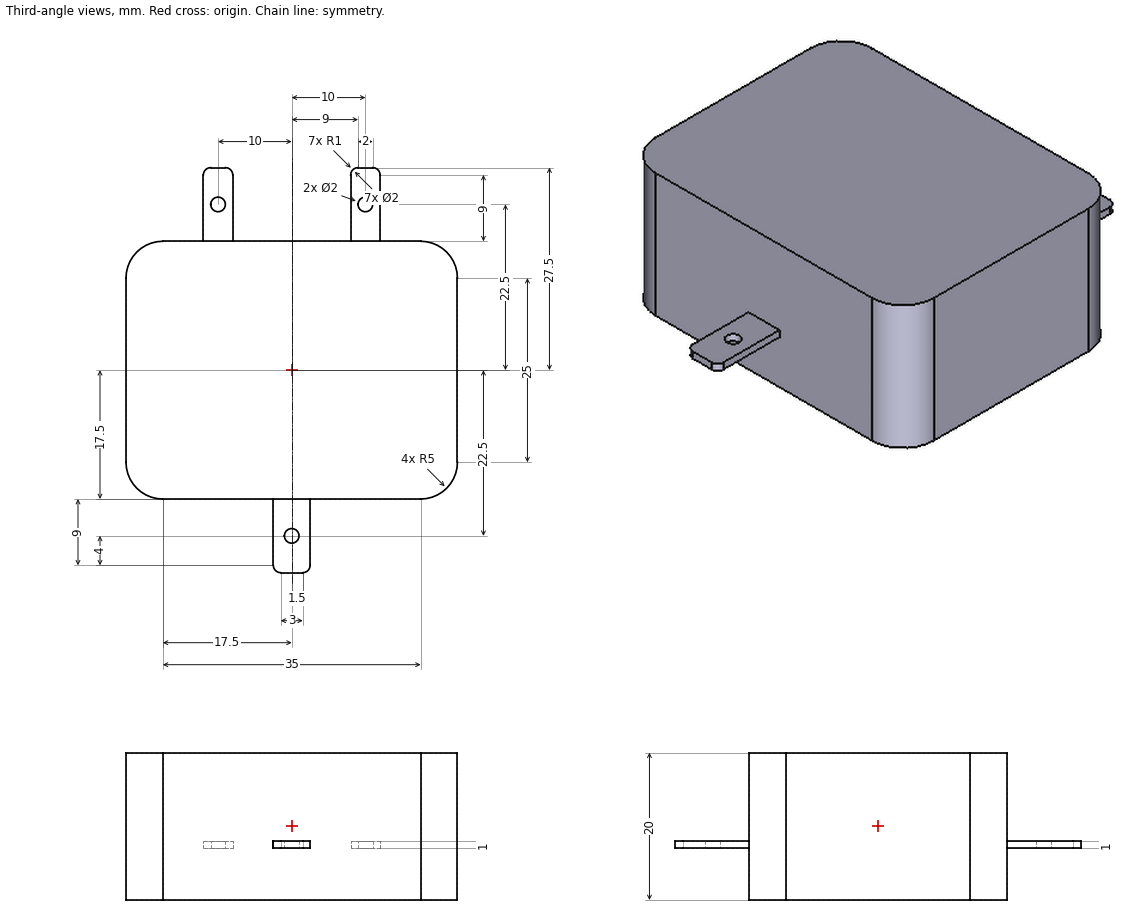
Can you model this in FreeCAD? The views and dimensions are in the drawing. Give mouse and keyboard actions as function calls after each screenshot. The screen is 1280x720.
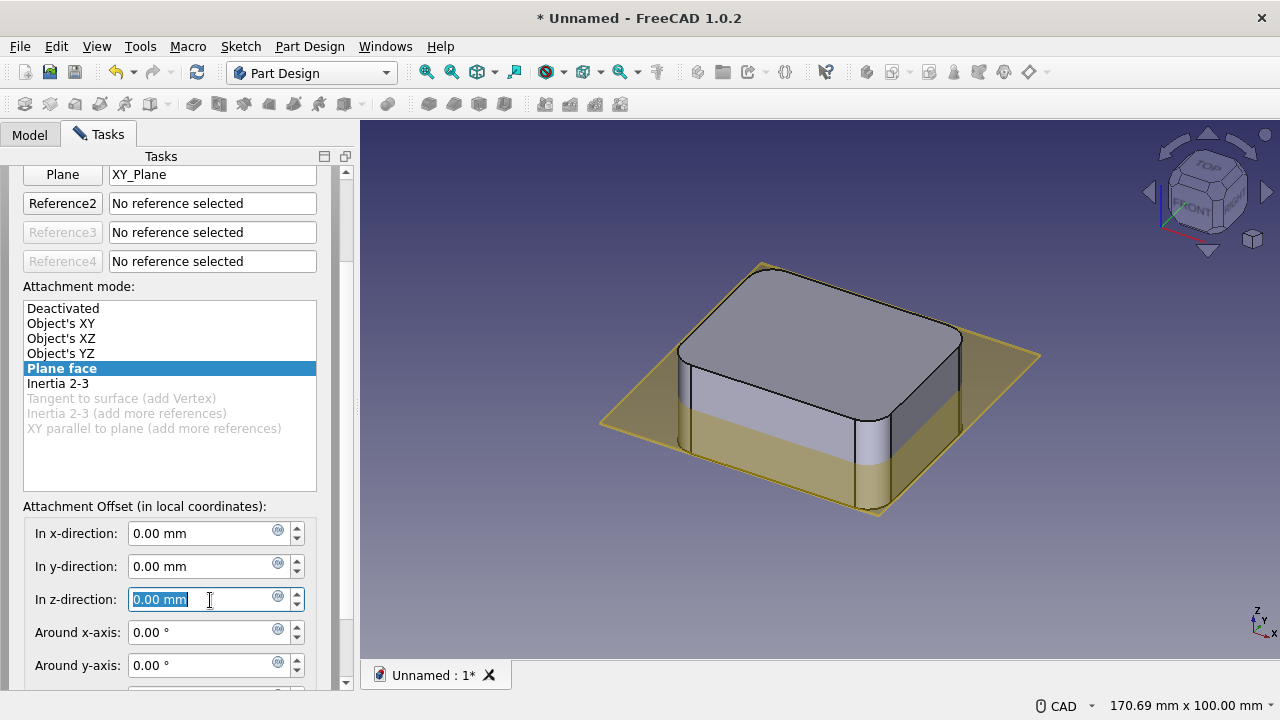
text(-3)
key(Tab)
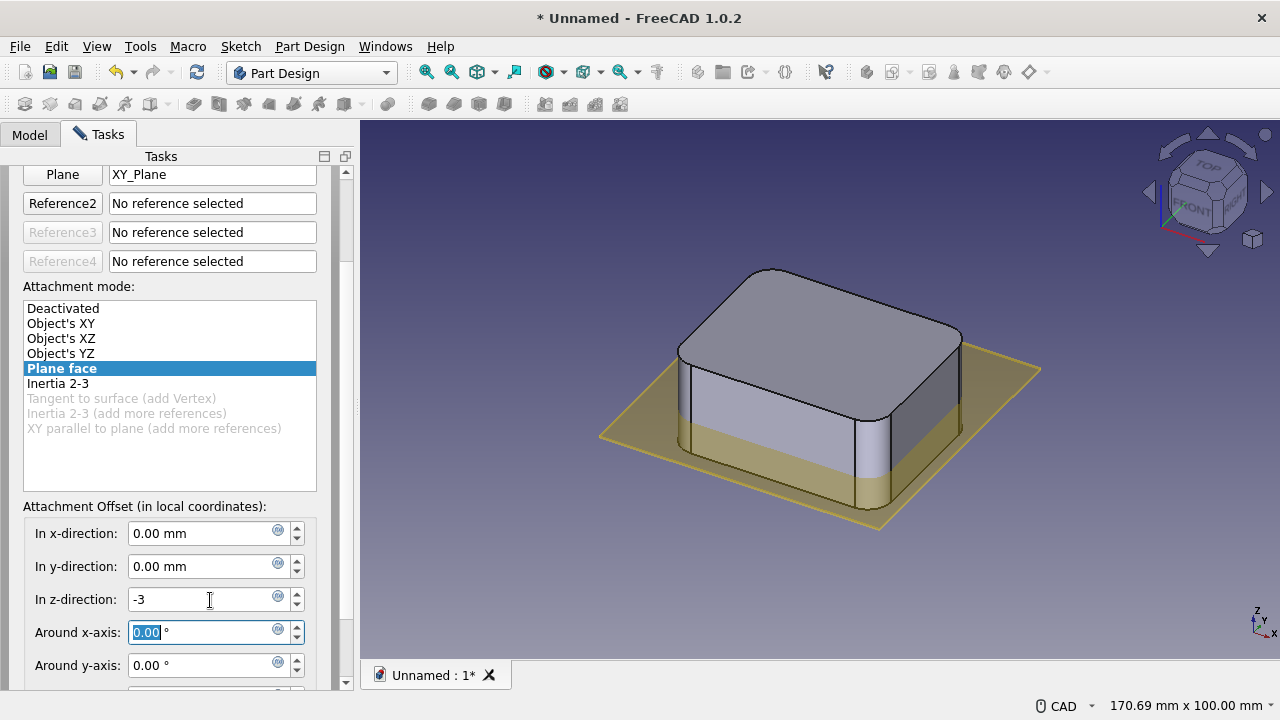
scroll(346, 428, up, 3)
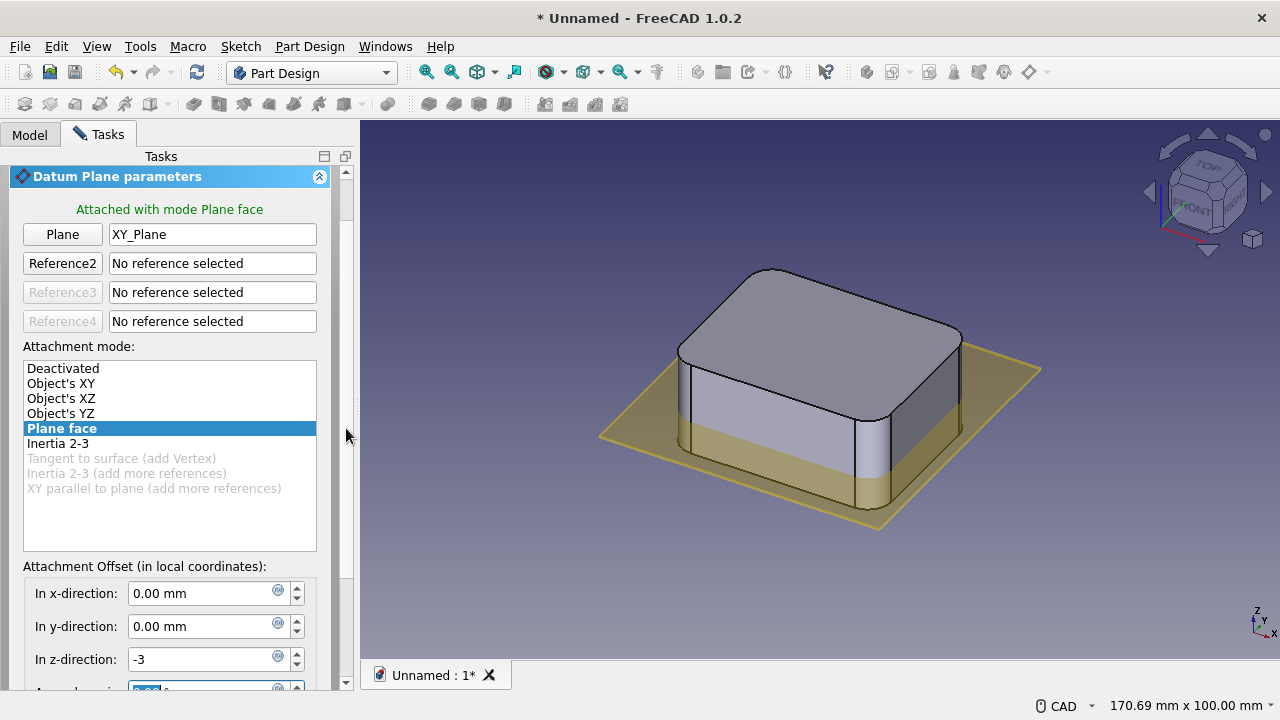
click(127, 195)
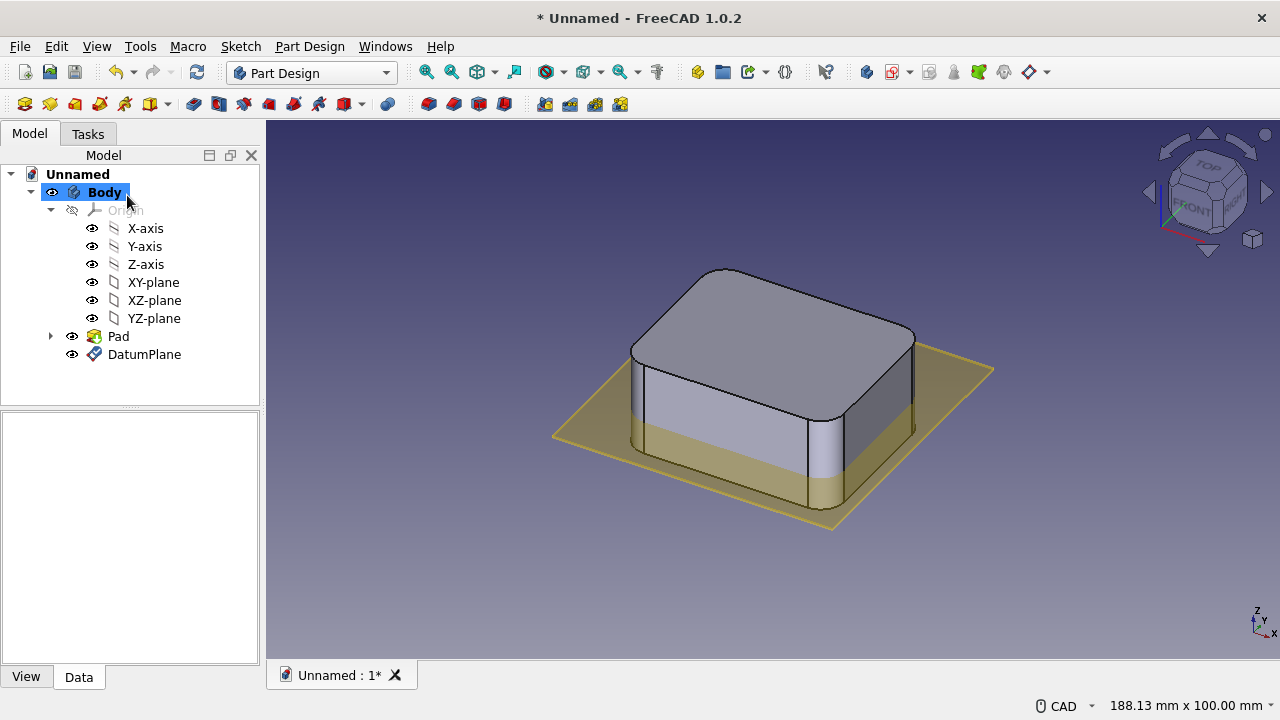
click(117, 354)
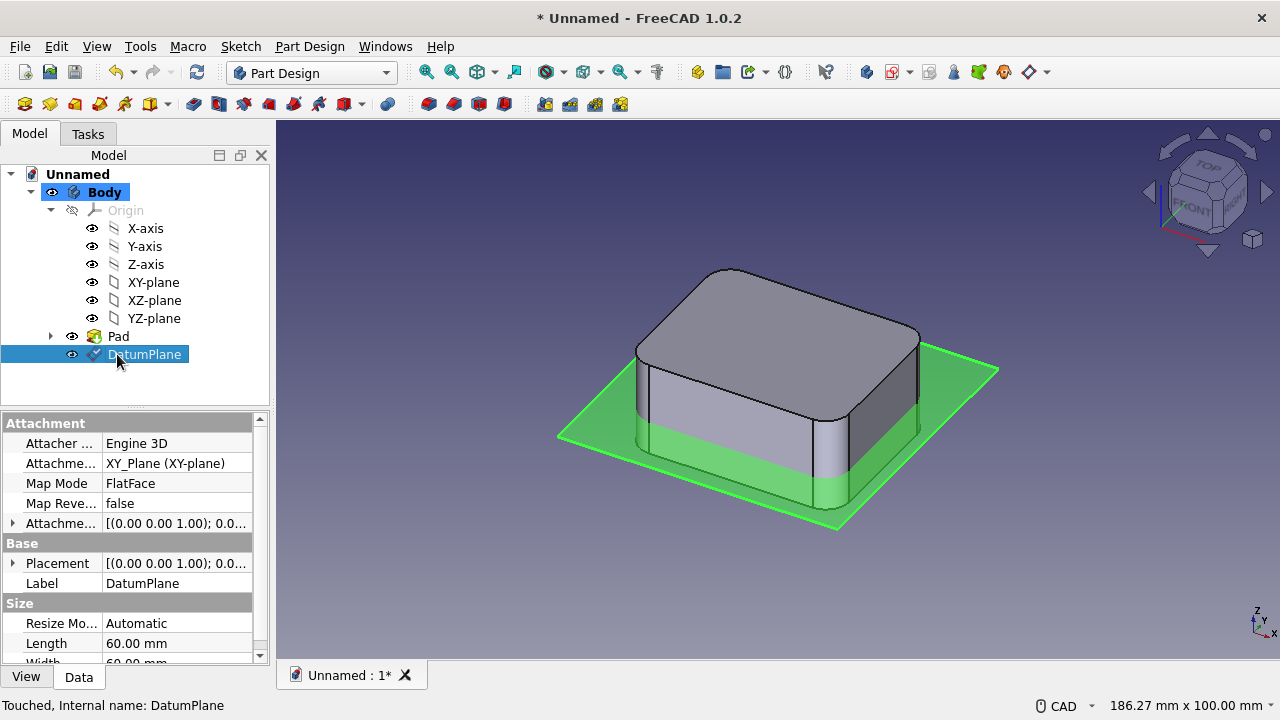
click(892, 72)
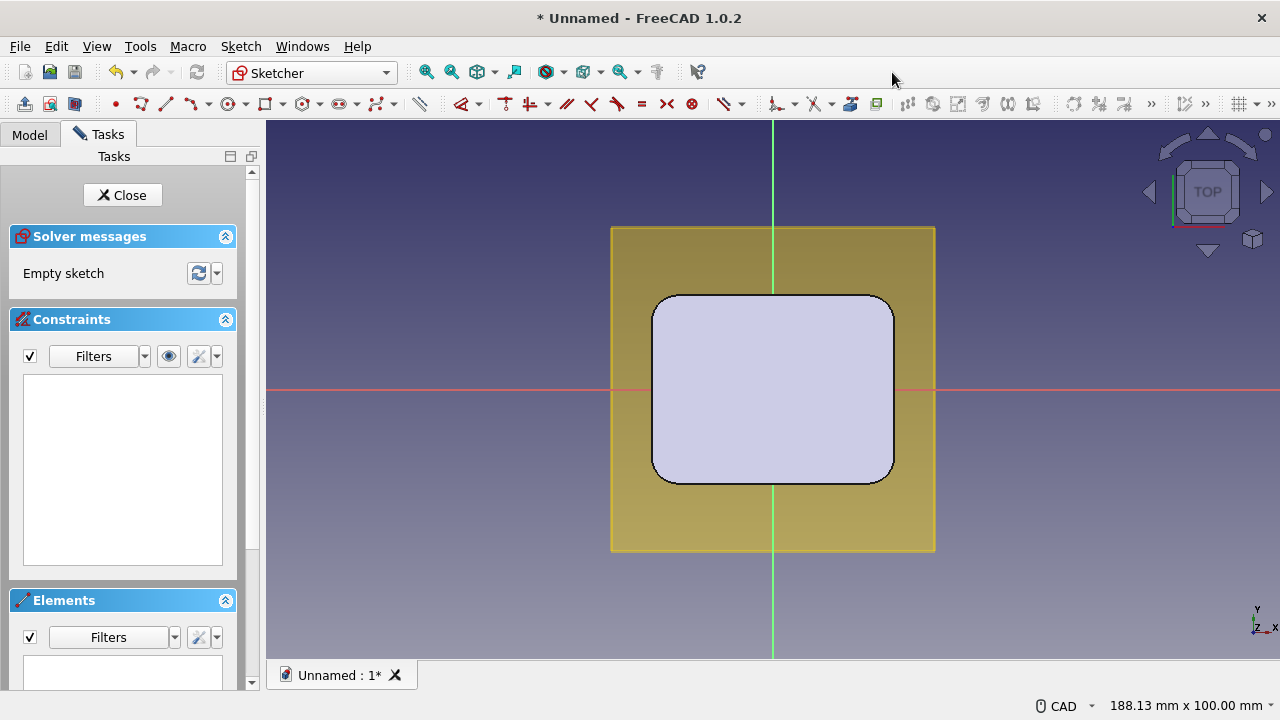
click(75, 104)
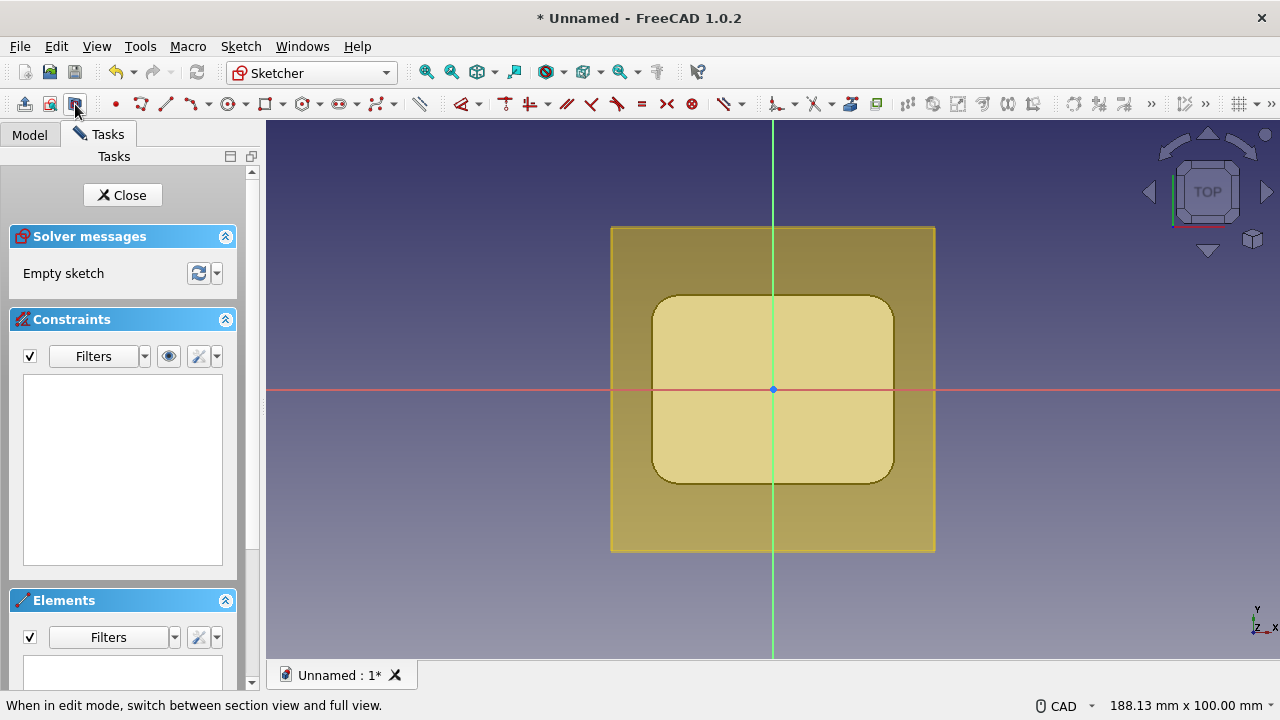
click(166, 104)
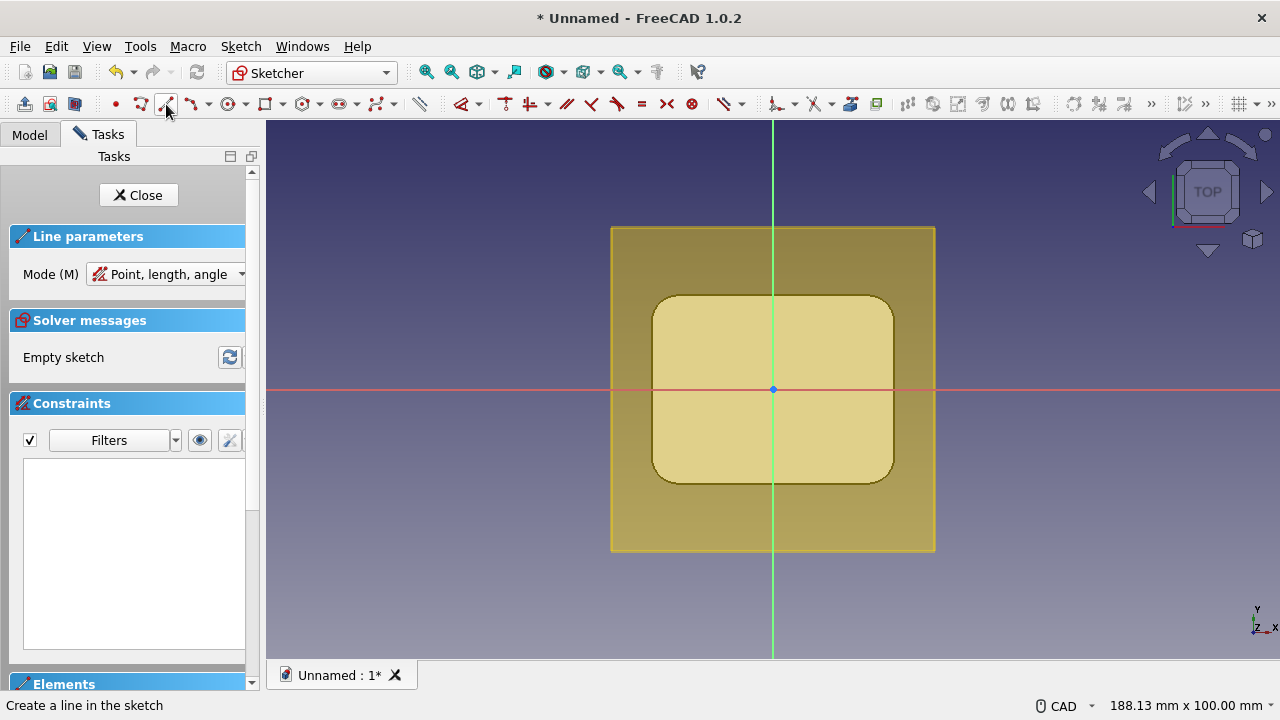
click(822, 241)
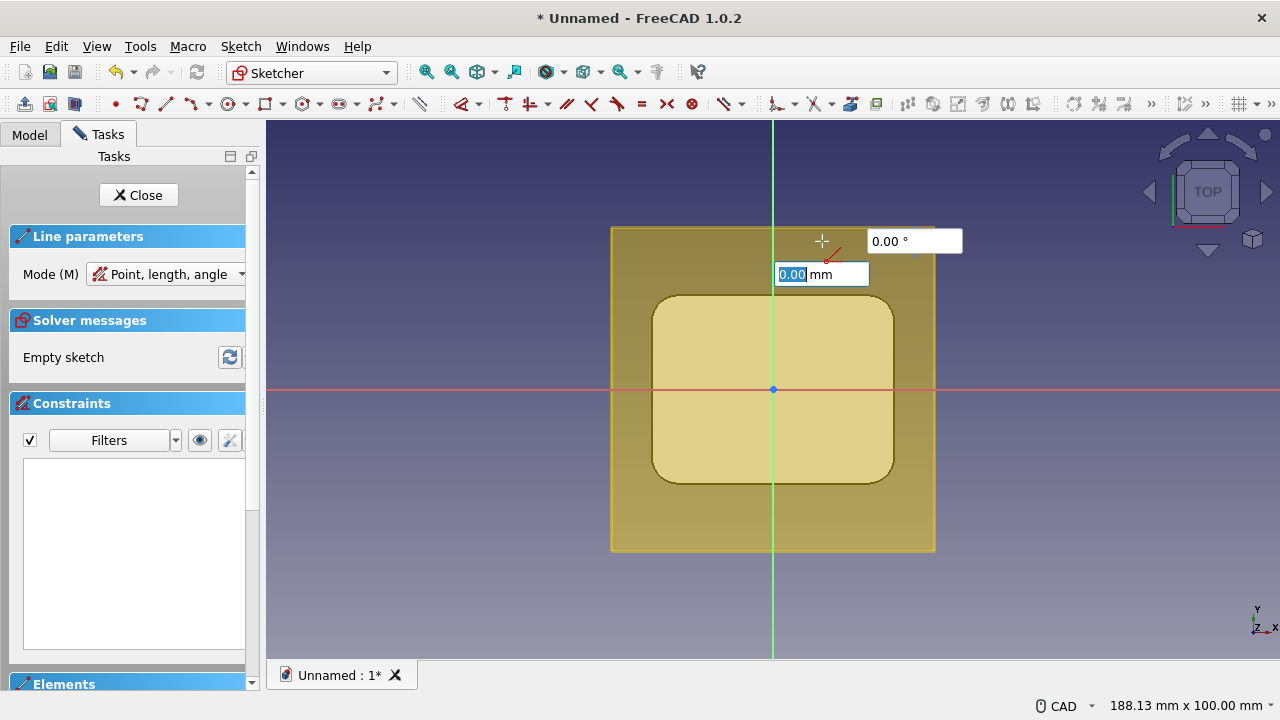
scroll(832, 241, up, 2)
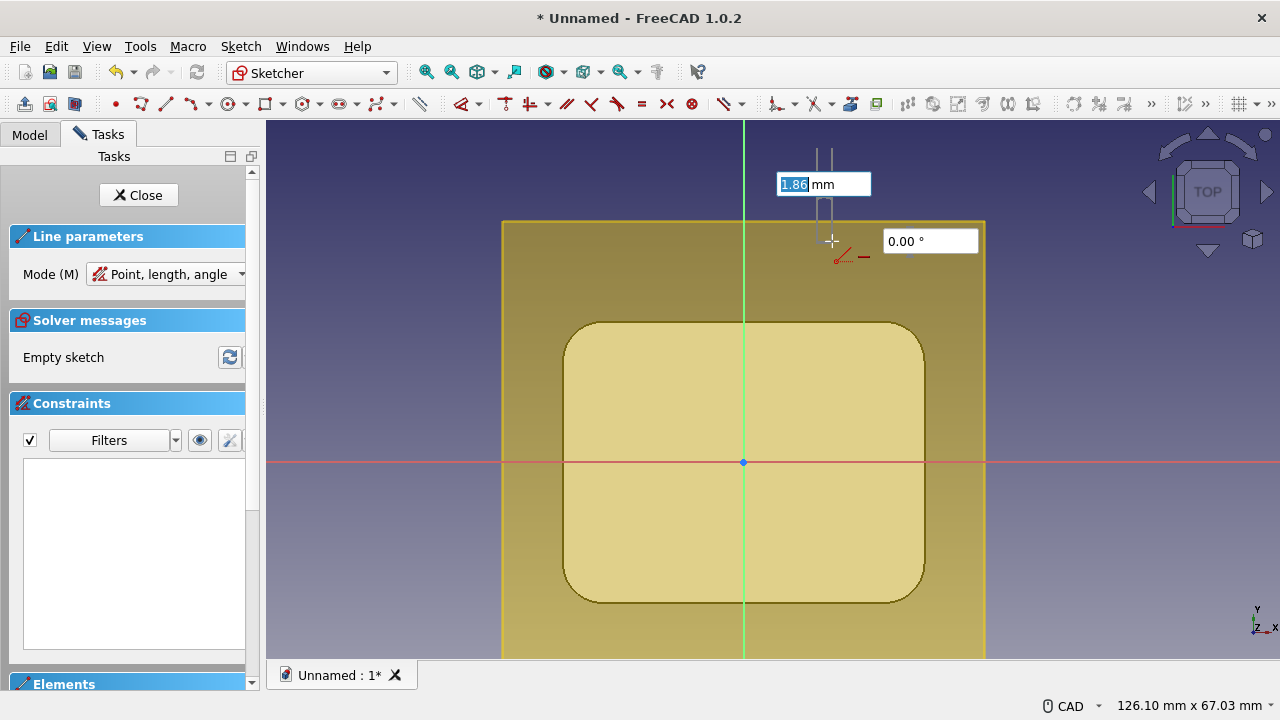
click(832, 241)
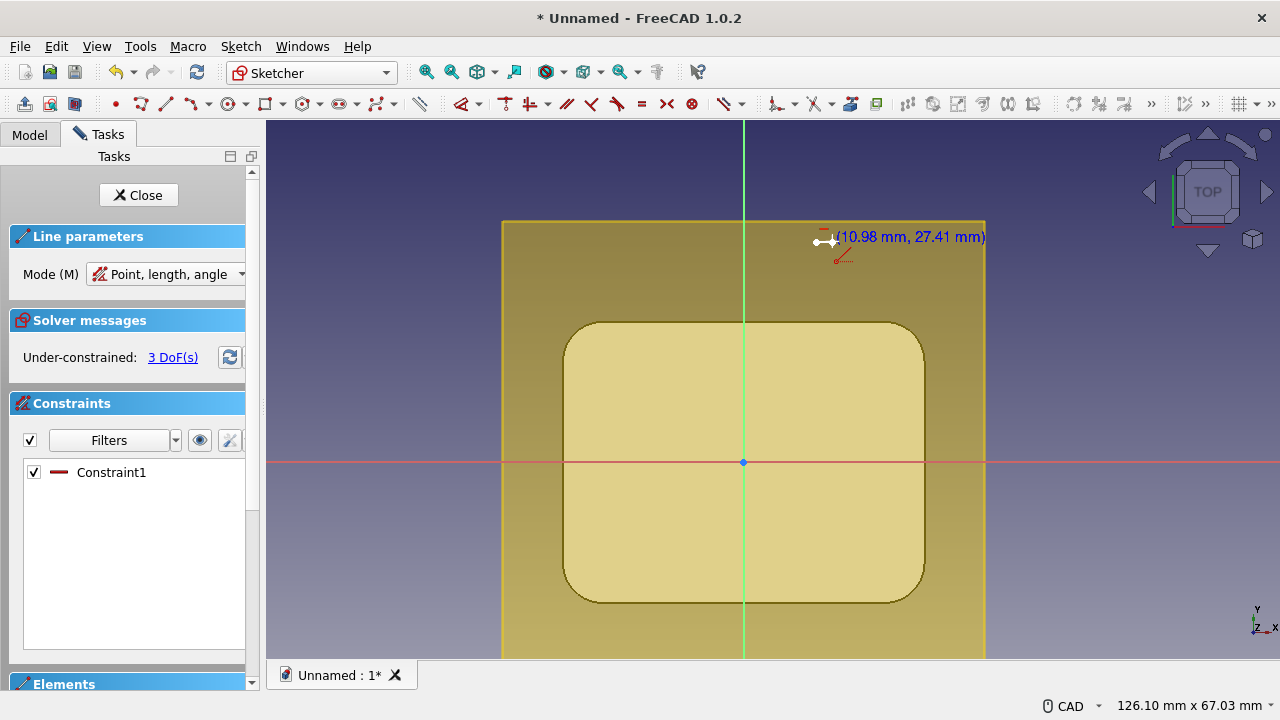
click(141, 104)